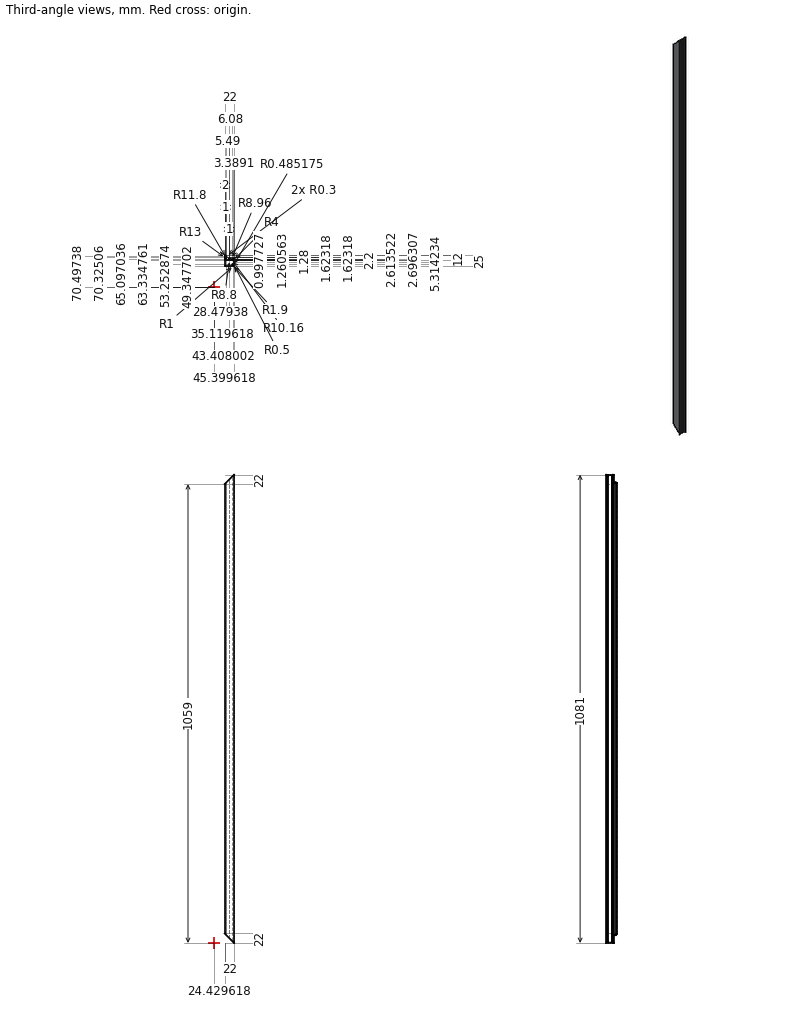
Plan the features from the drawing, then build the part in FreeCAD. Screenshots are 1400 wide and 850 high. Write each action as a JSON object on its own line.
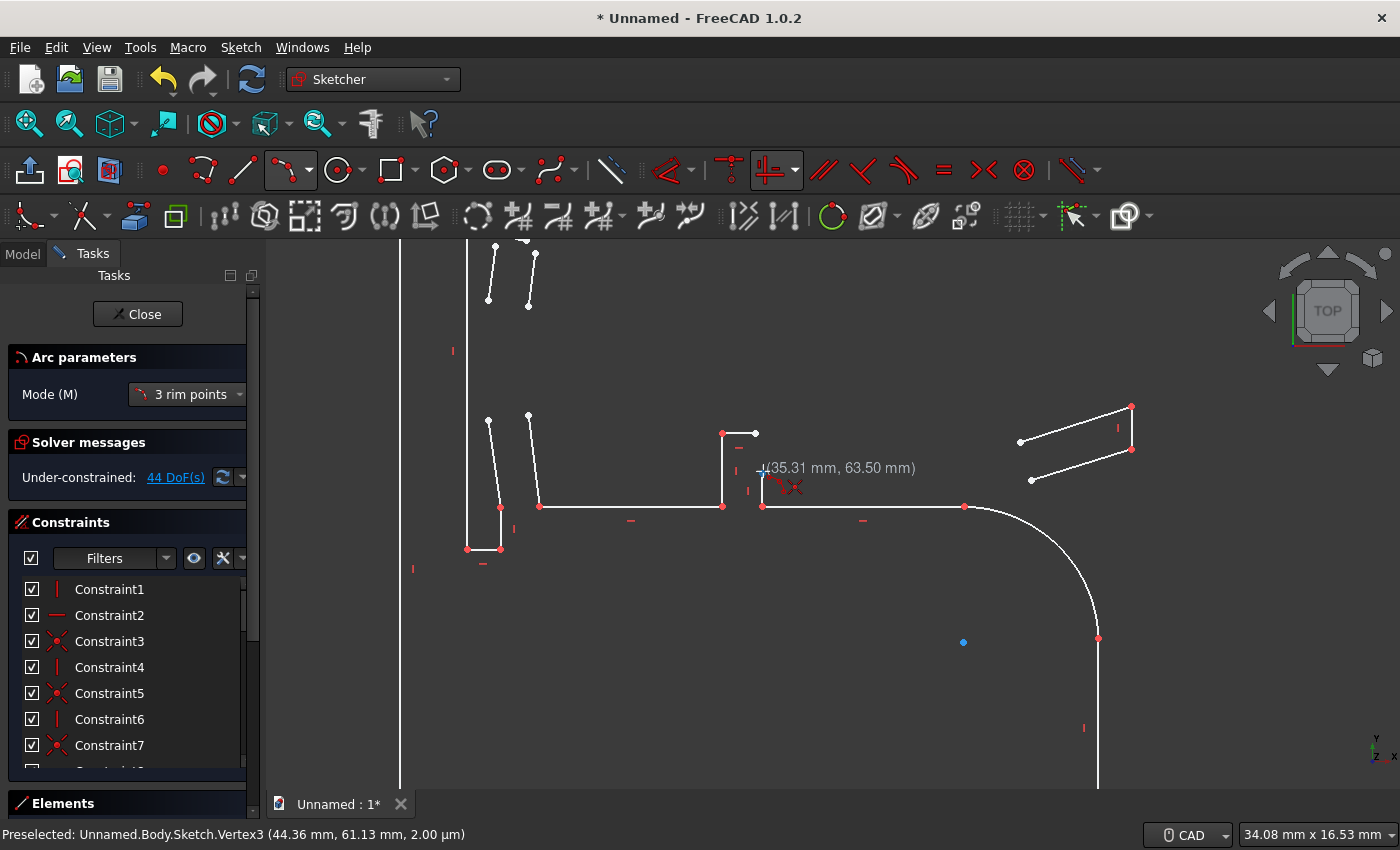
{"action": "left_click", "coordinate": [762, 474]}
{"action": "left_click", "coordinate": [836, 482]}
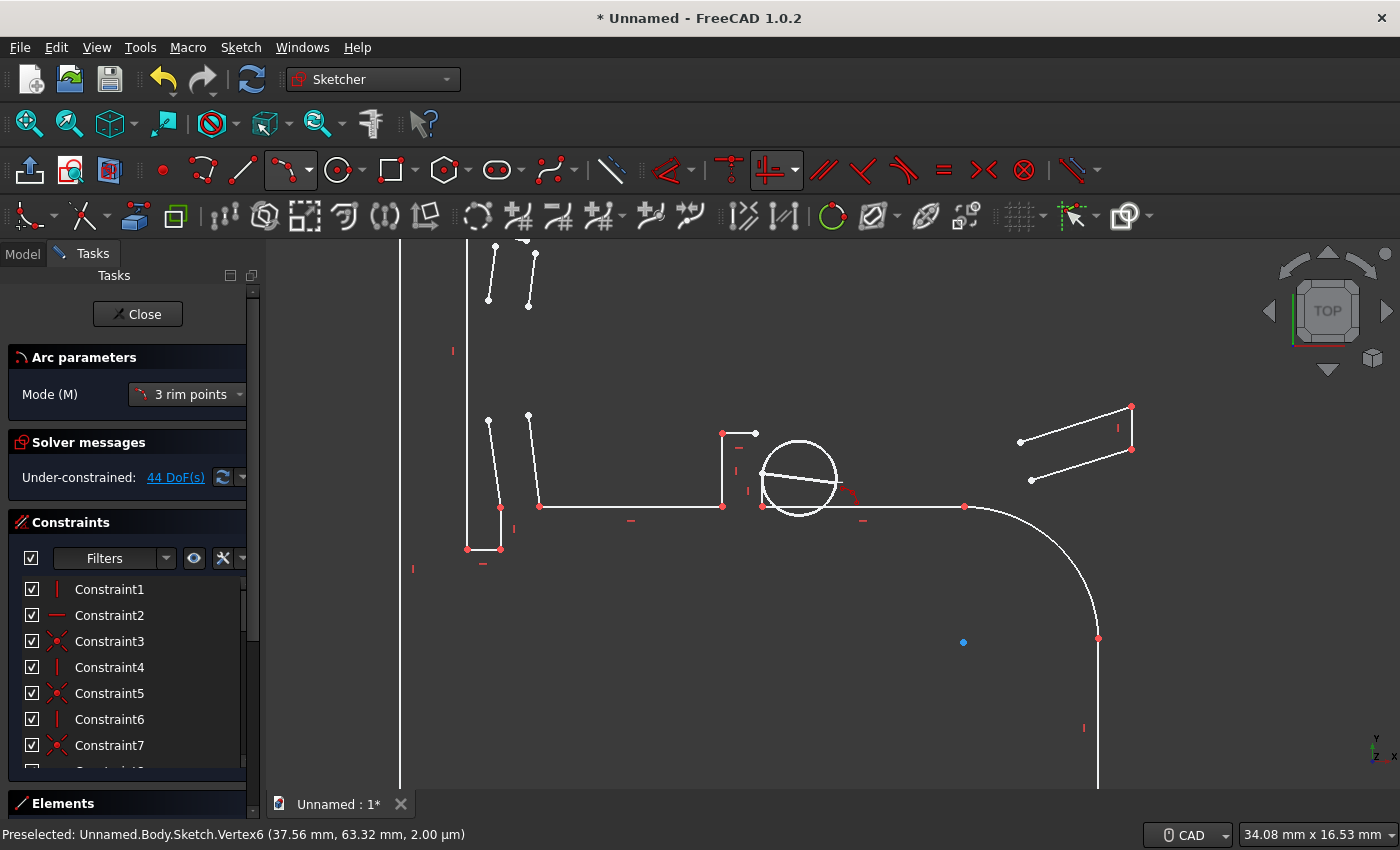
{"action": "scroll", "coordinate": [800, 474], "scroll_direction": "up", "scroll_amount": 10}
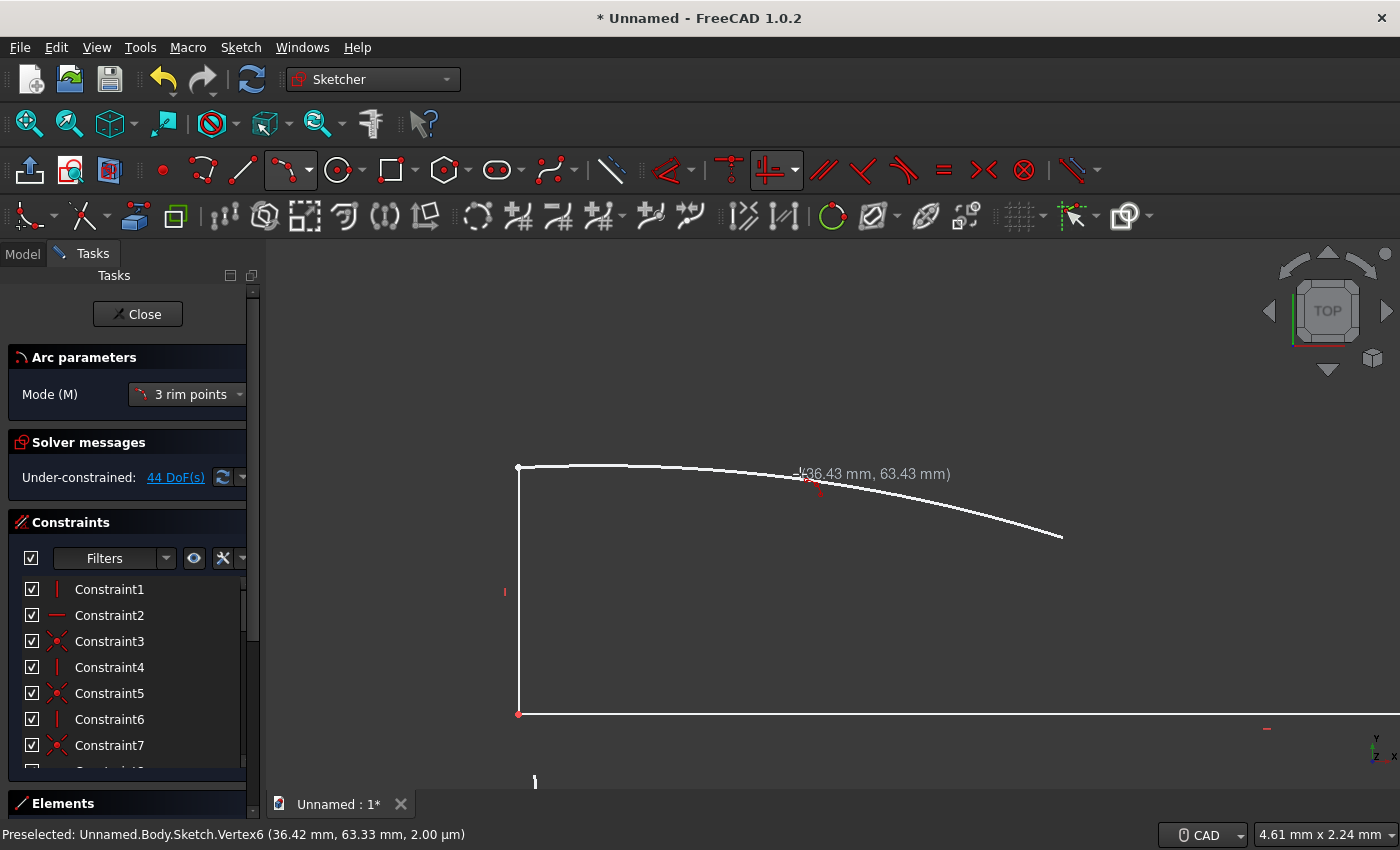
{"action": "left_click", "coordinate": [797, 470]}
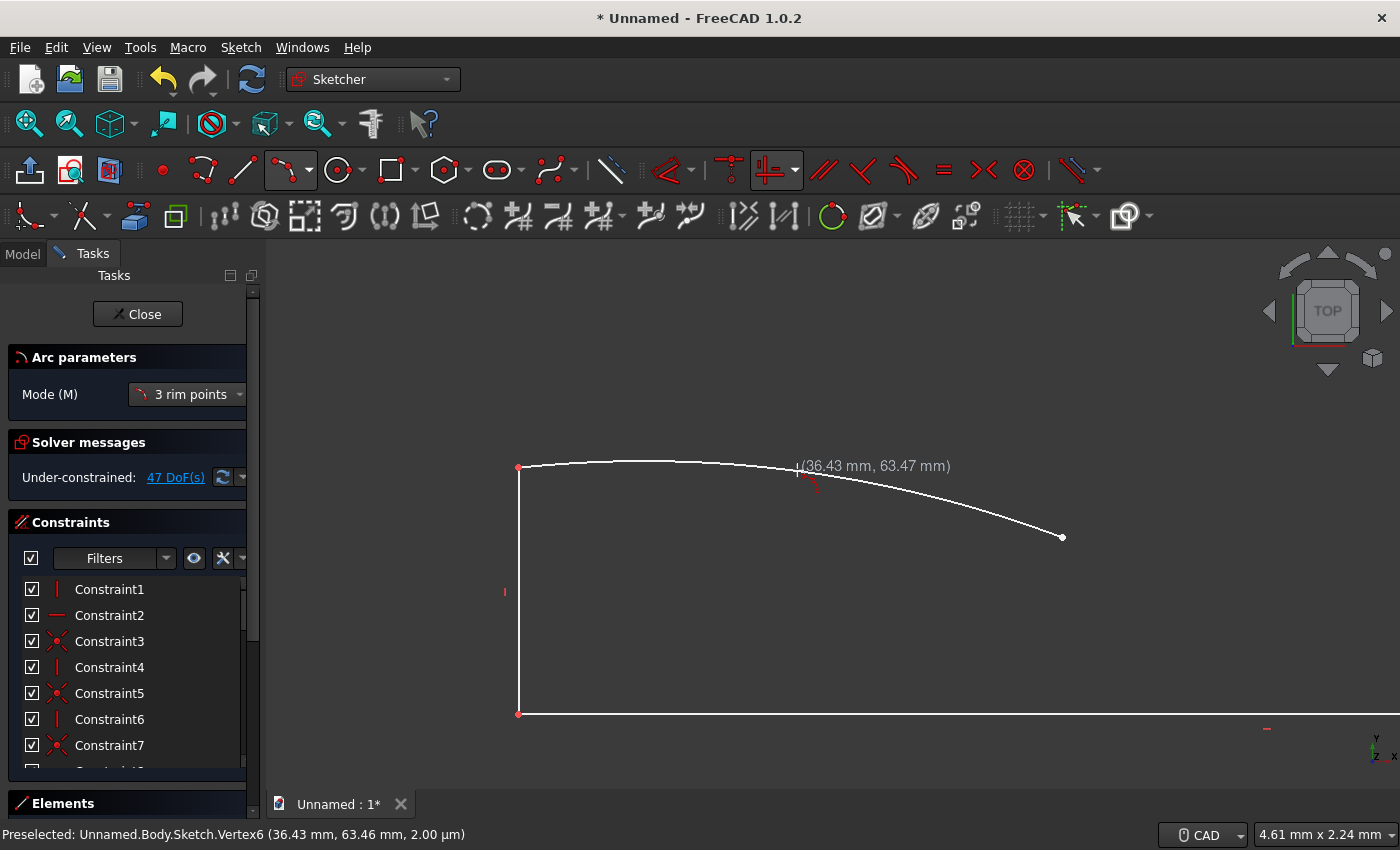
{"action": "scroll", "coordinate": [778, 473], "scroll_direction": "down", "scroll_amount": 14}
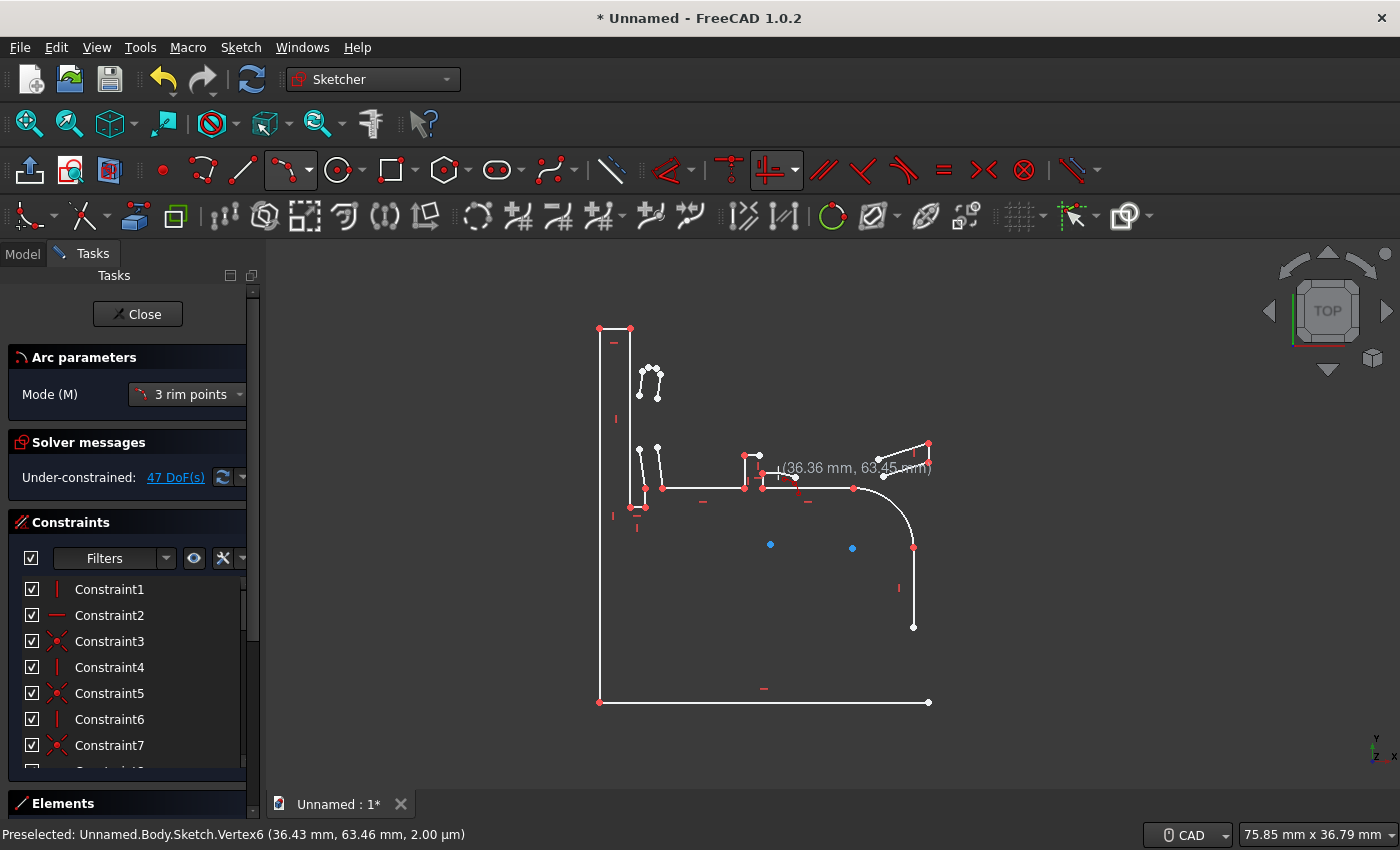
{"action": "scroll", "coordinate": [796, 477], "scroll_direction": "up", "scroll_amount": 3}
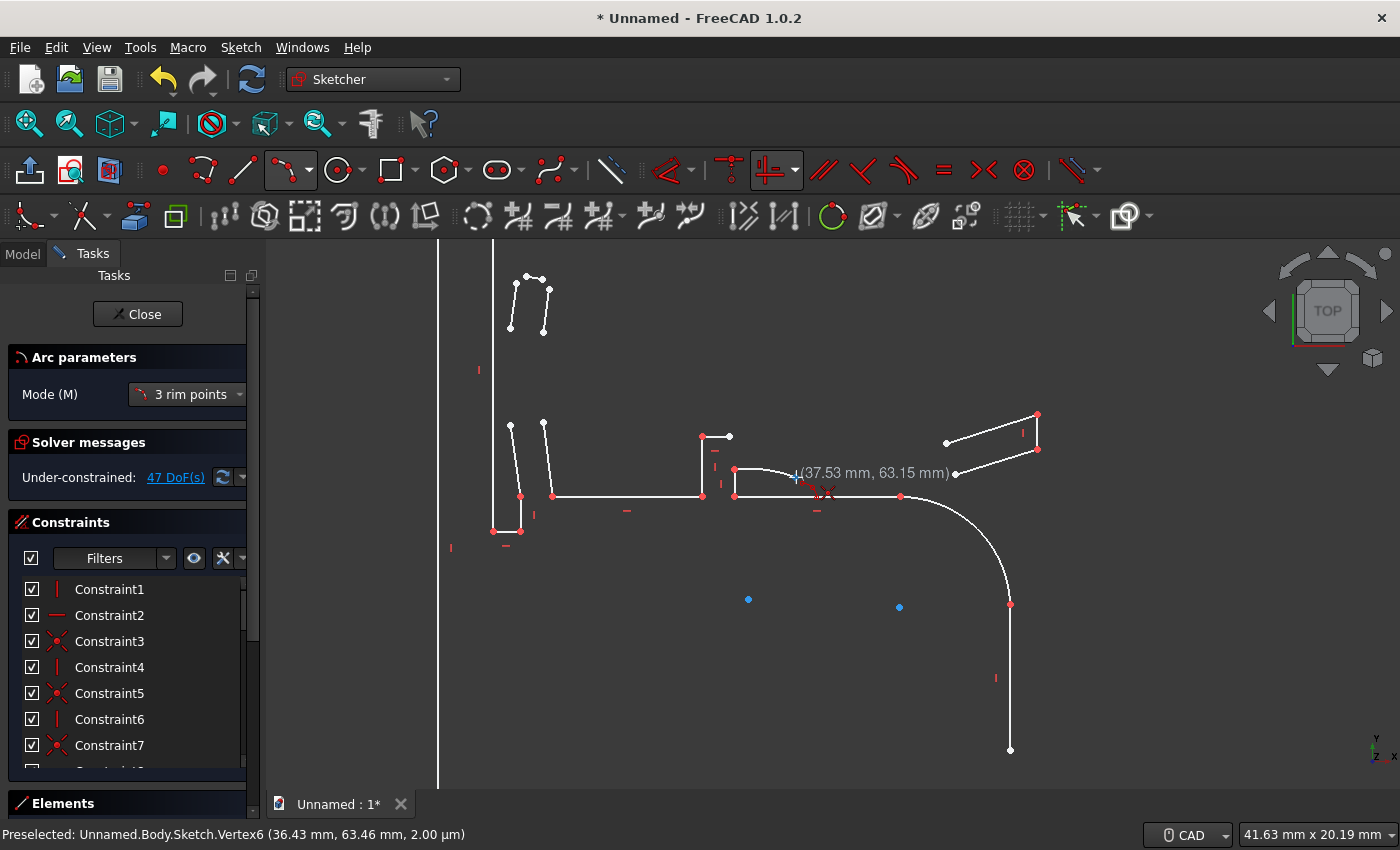
{"action": "left_click", "coordinate": [795, 477]}
{"action": "left_click", "coordinate": [955, 475]}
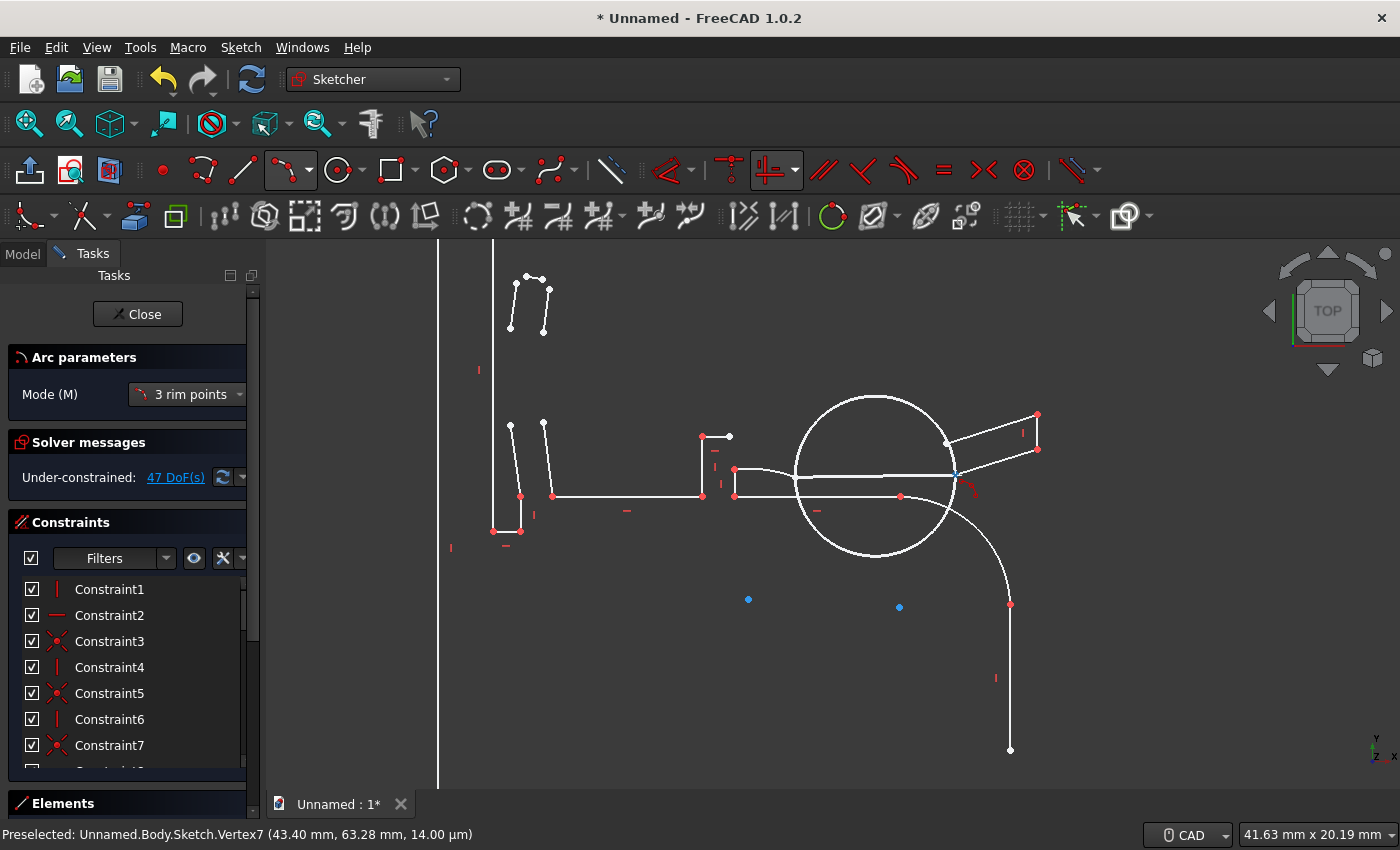
{"action": "scroll", "coordinate": [908, 484], "scroll_direction": "up", "scroll_amount": 3}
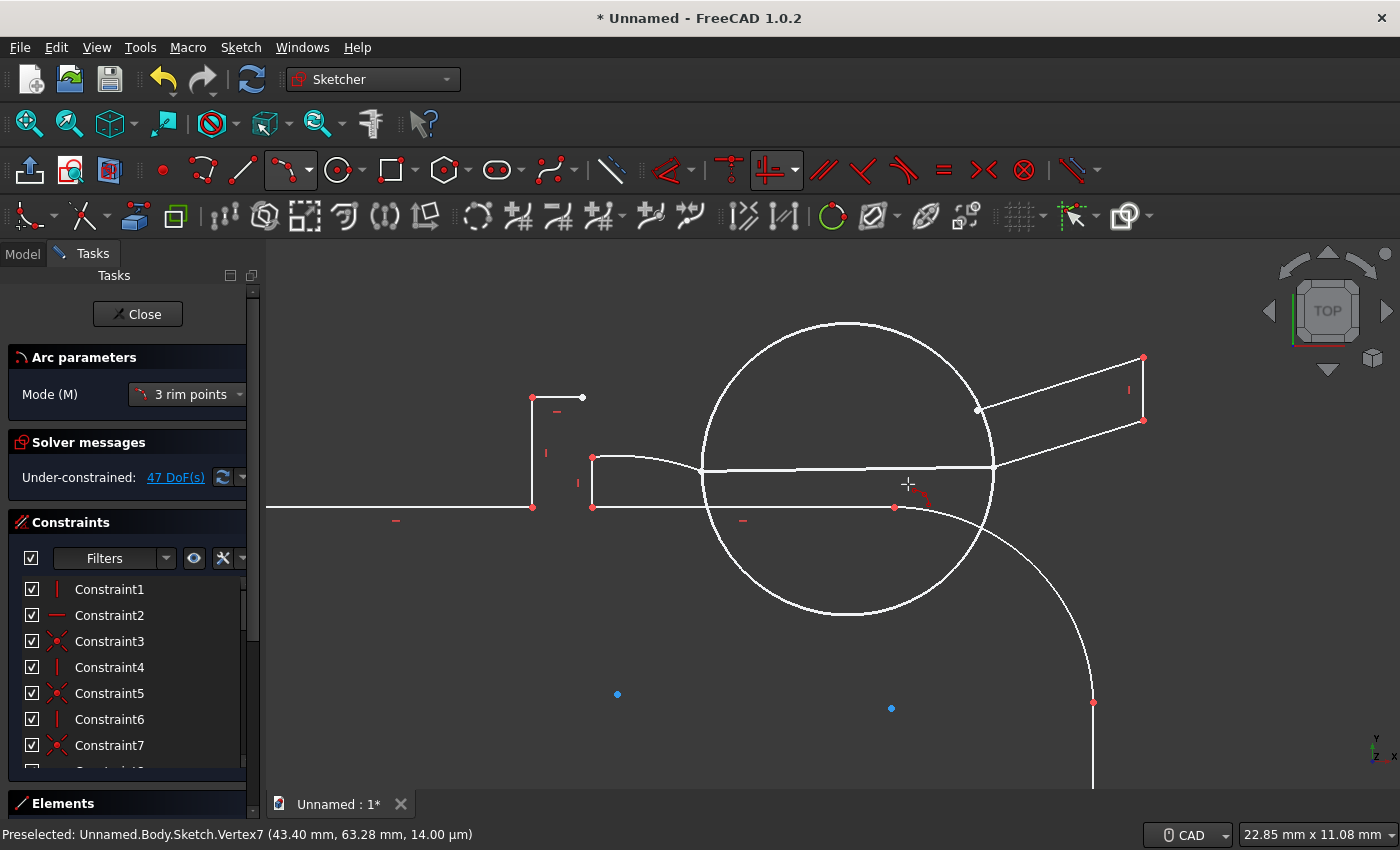
{"action": "left_click", "coordinate": [908, 484]}